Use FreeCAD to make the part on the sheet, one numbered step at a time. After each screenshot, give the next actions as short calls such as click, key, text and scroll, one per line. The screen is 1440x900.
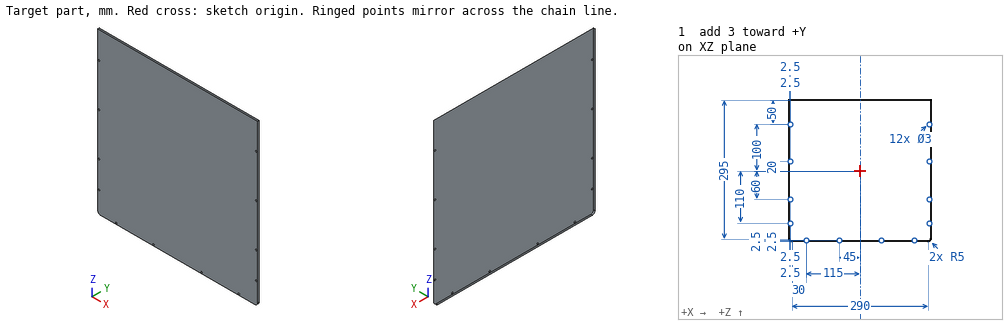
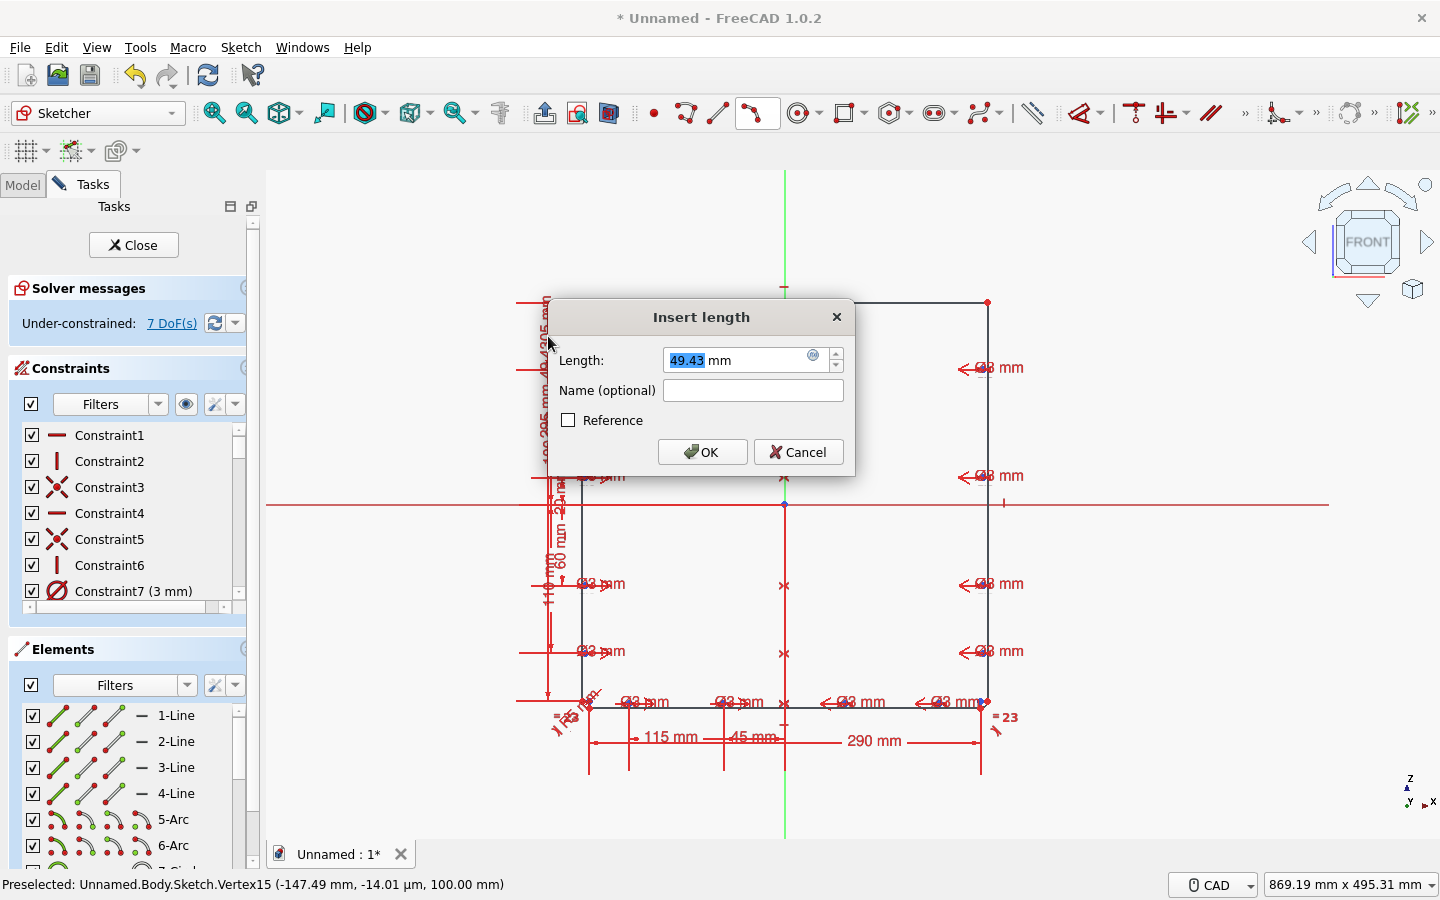
text(50)
key(Return)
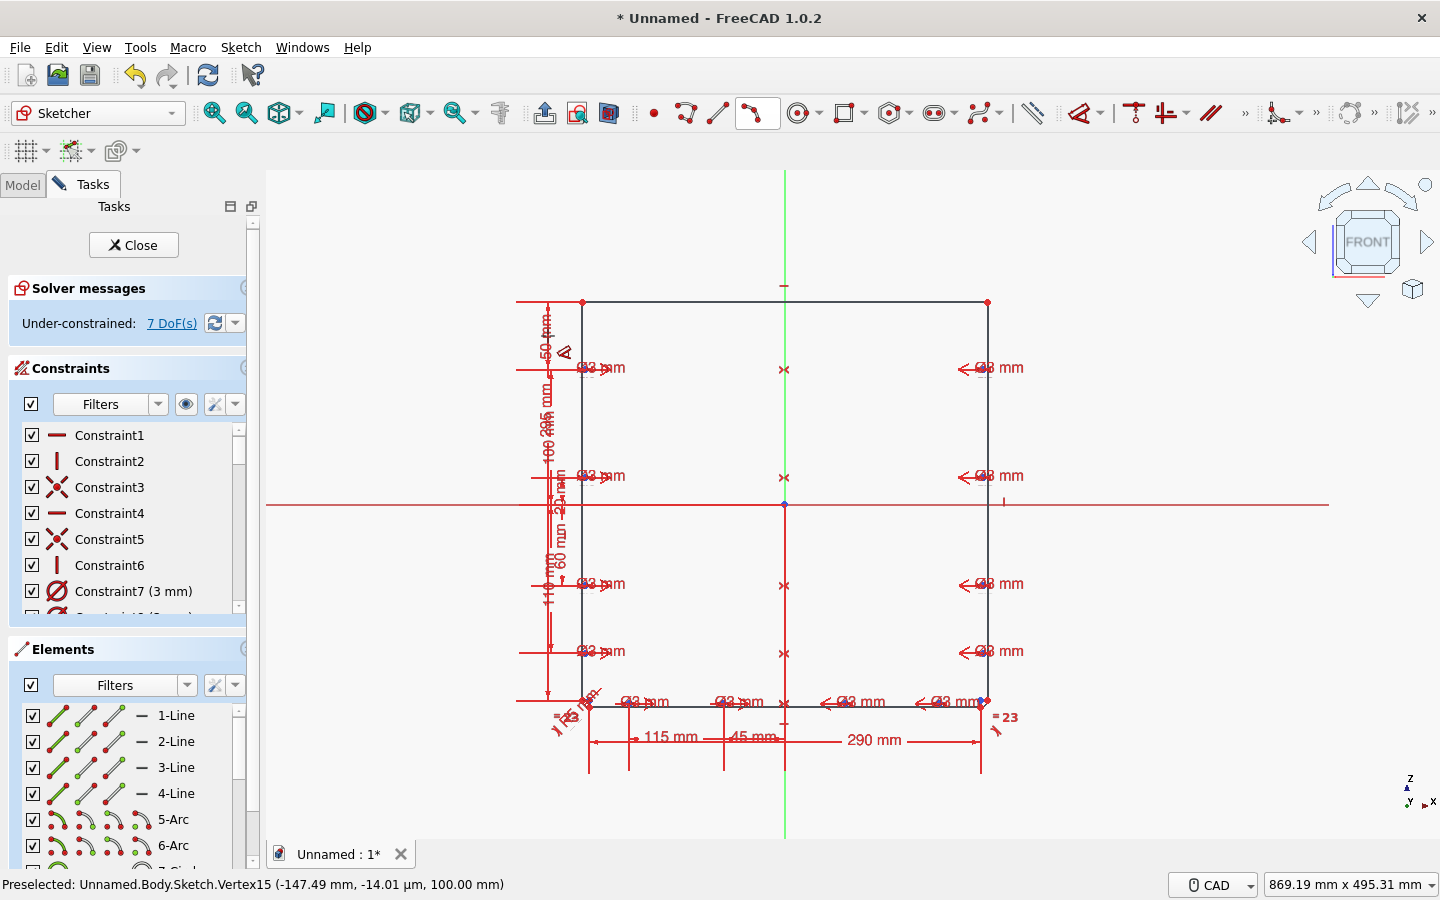
scroll(589, 707, up, 3)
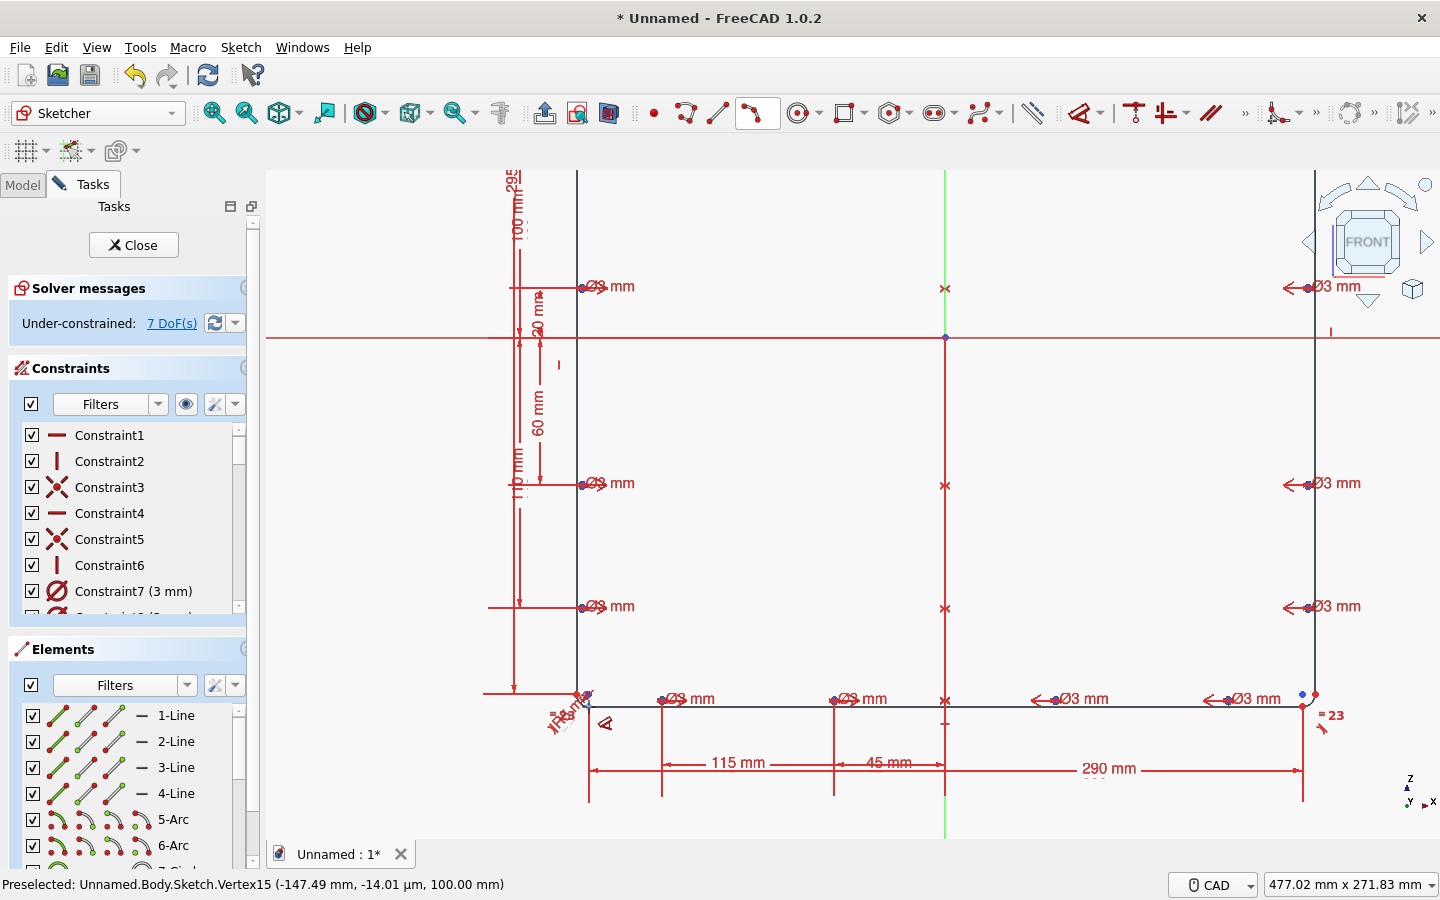
click(589, 707)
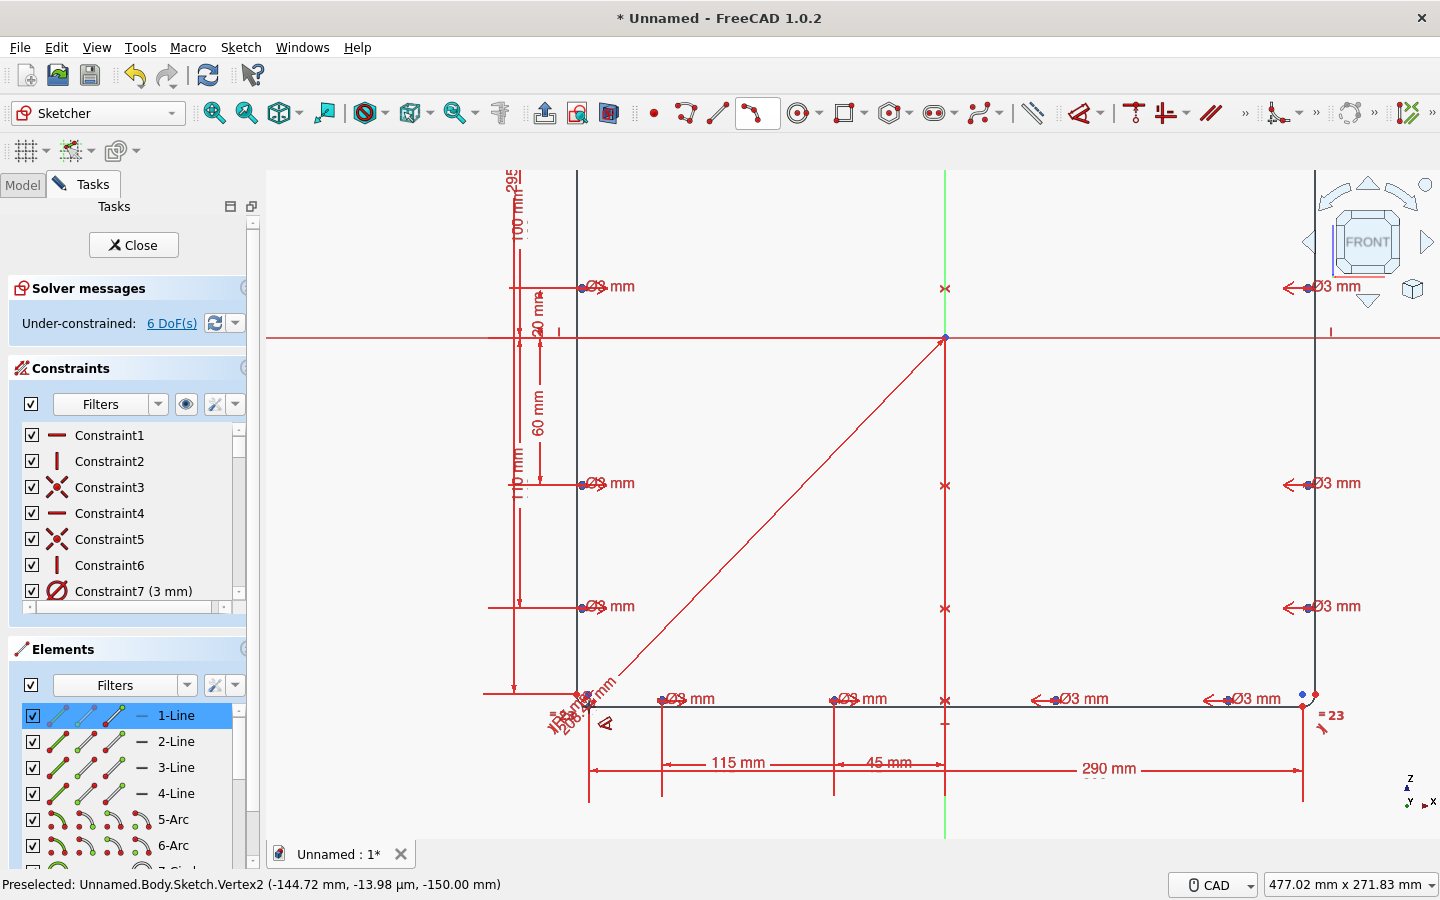
click(662, 701)
click(626, 741)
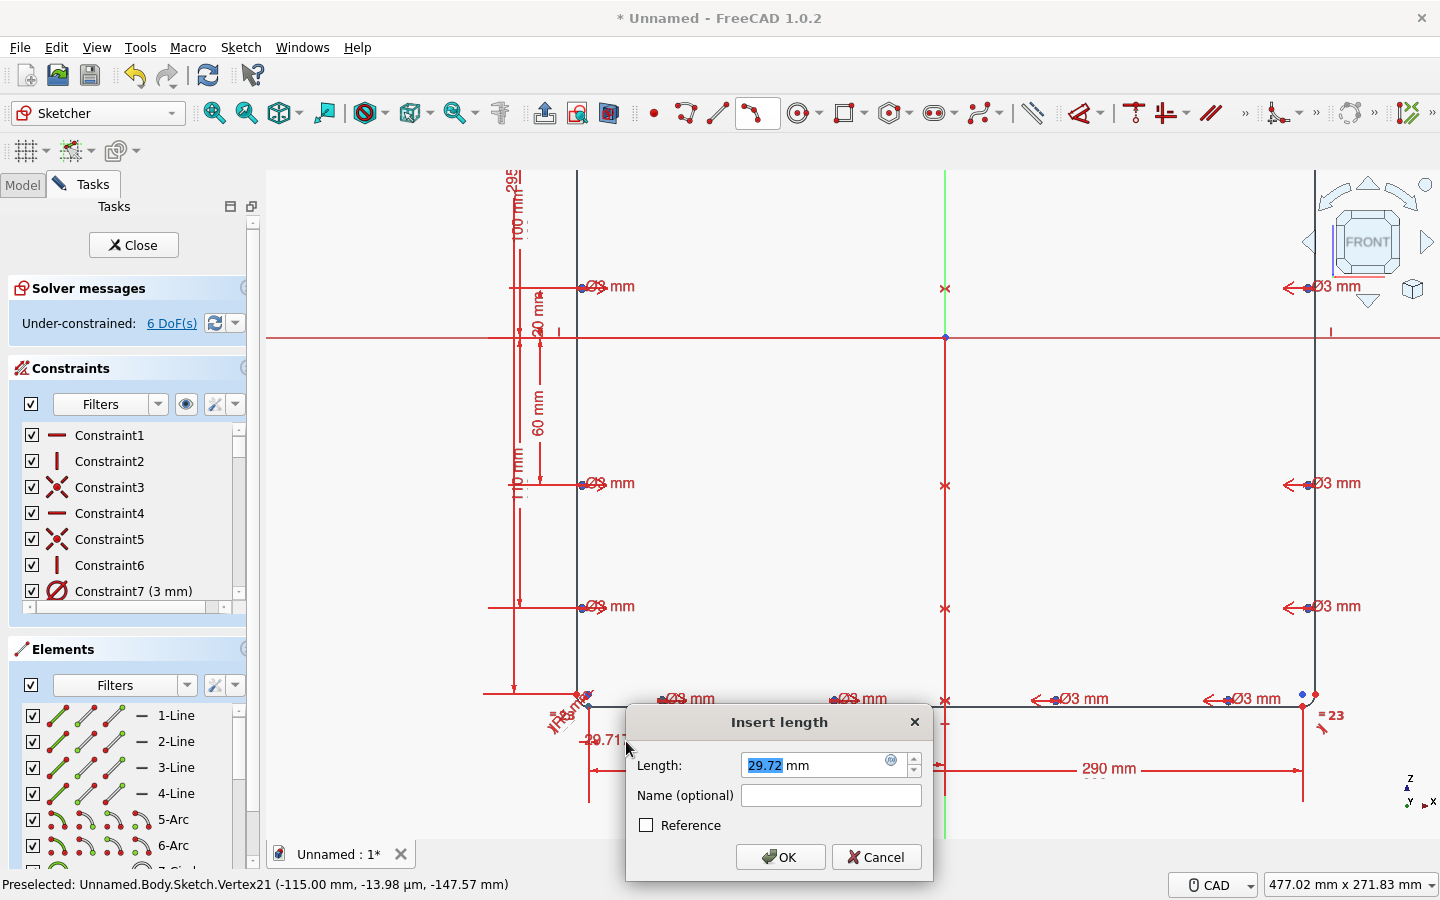
text(30)
key(Return)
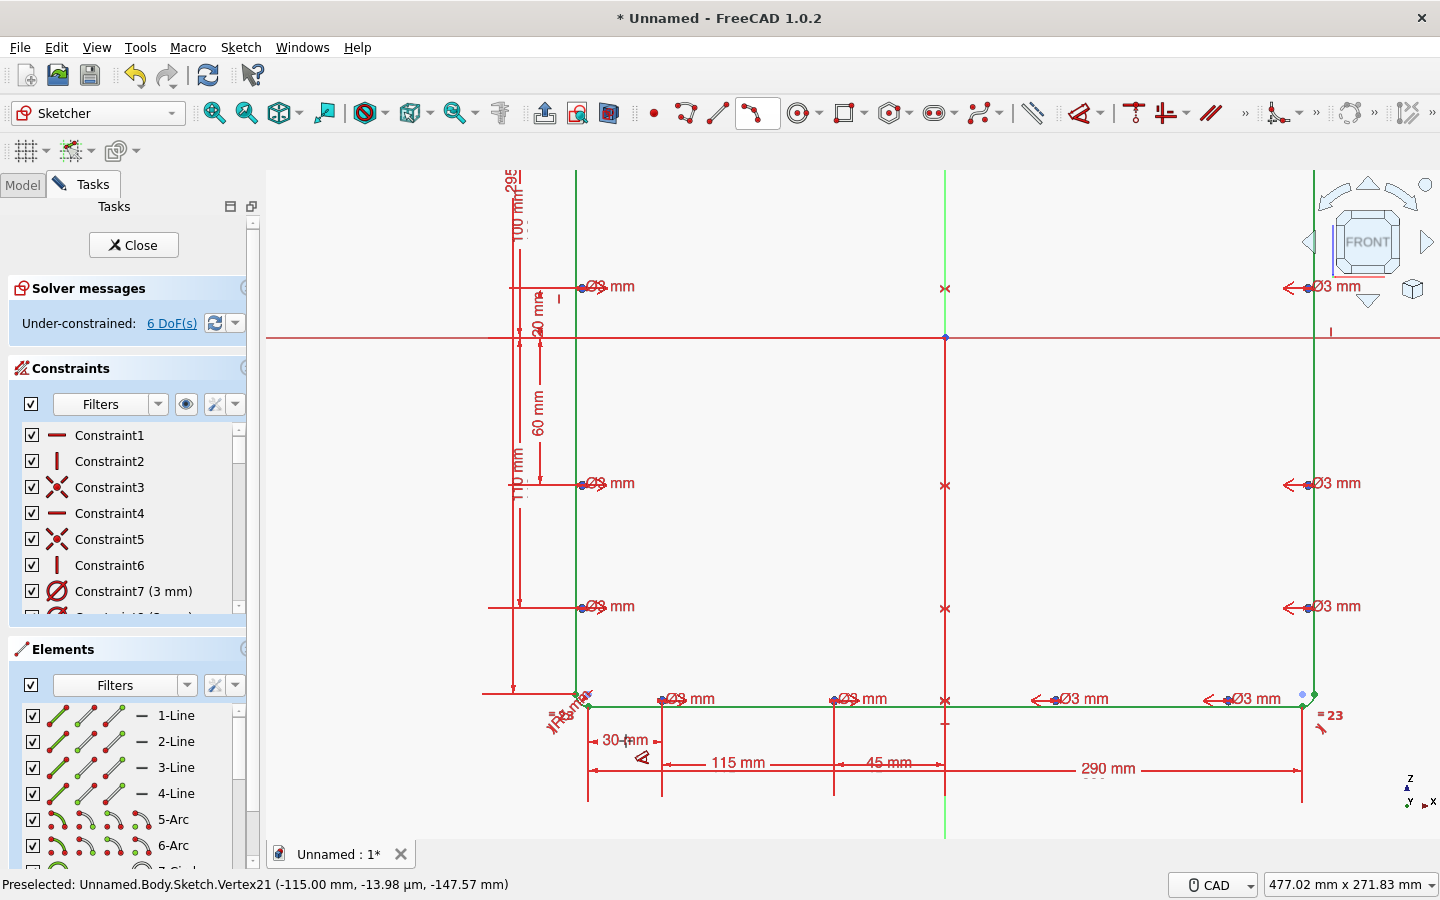
scroll(589, 707, down, 3)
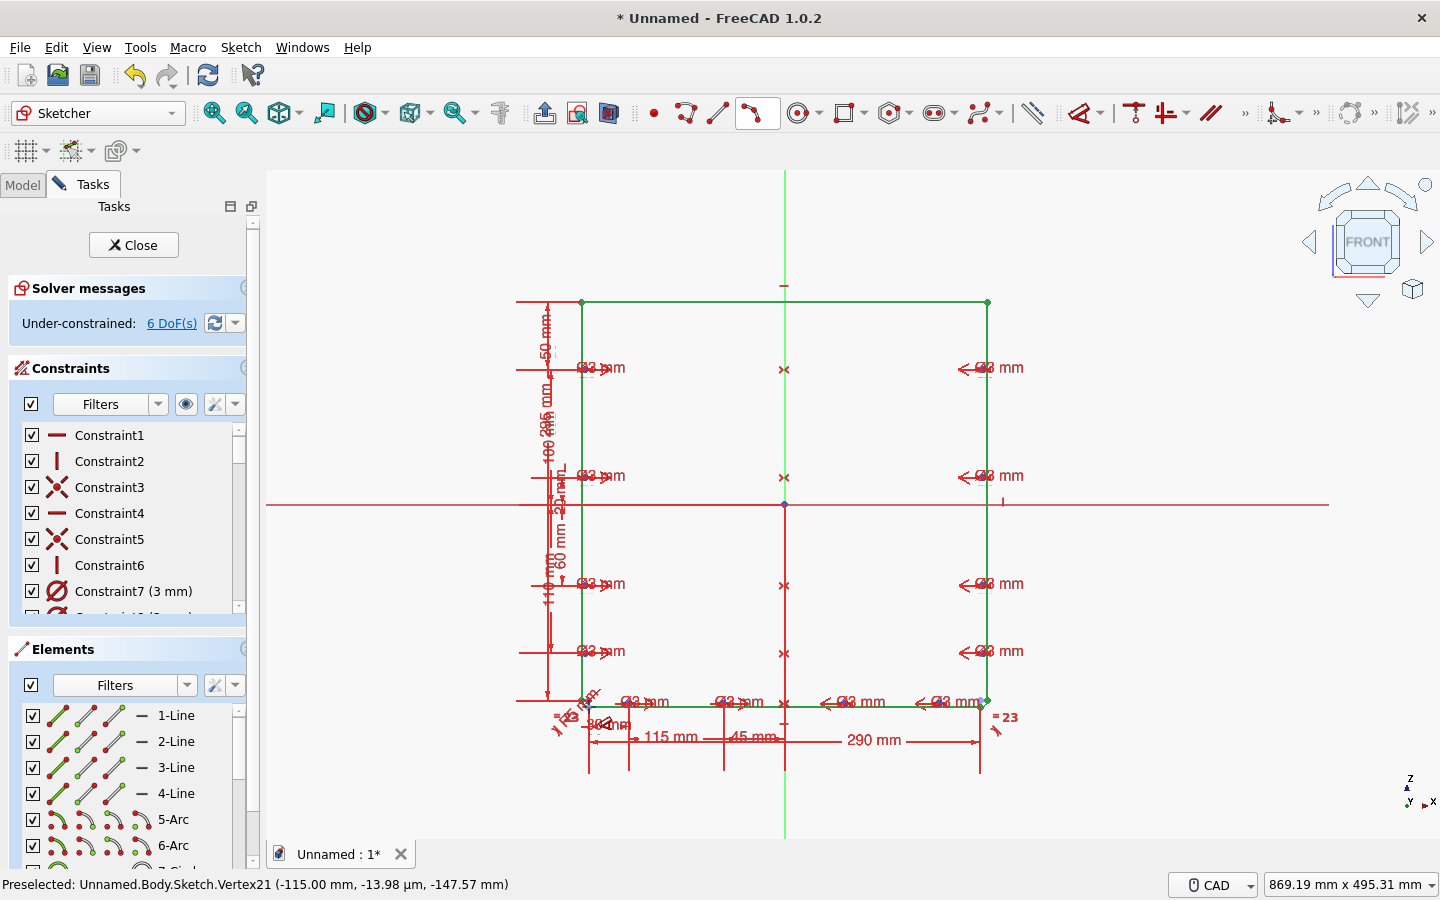
scroll(582, 302, up, 13)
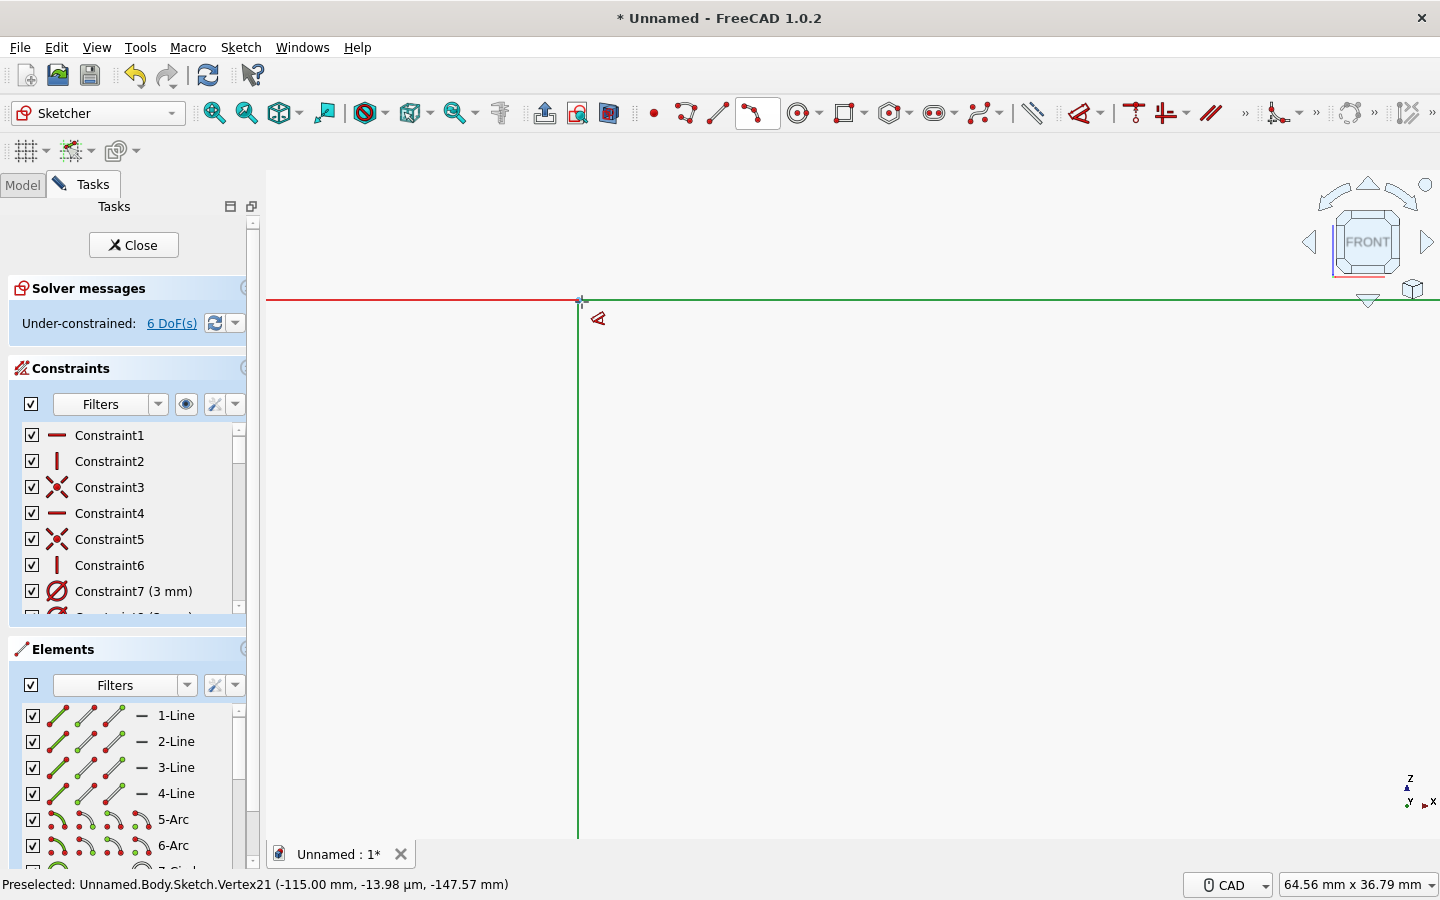
click(578, 300)